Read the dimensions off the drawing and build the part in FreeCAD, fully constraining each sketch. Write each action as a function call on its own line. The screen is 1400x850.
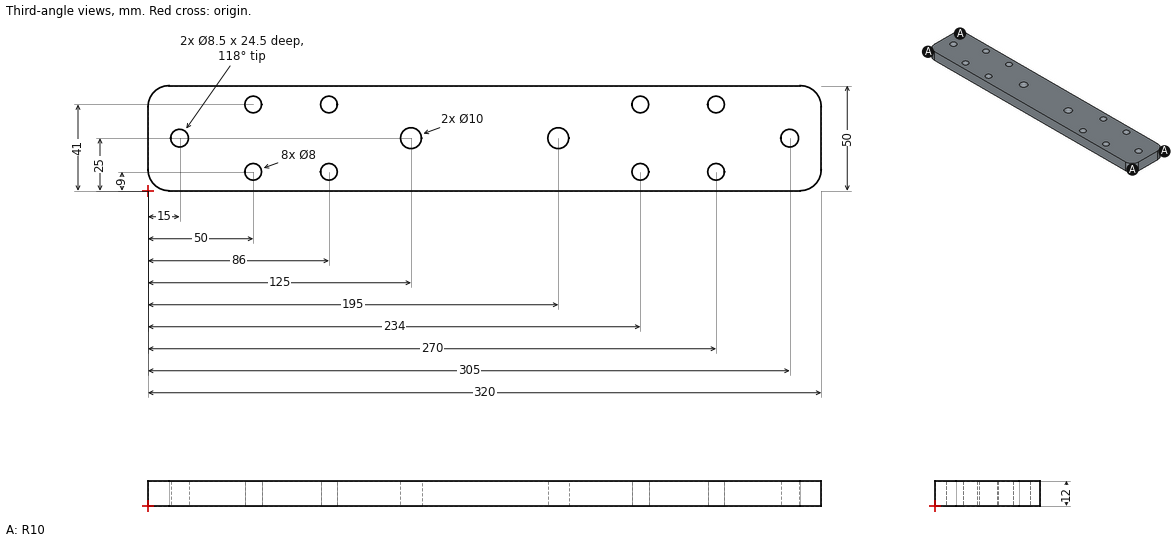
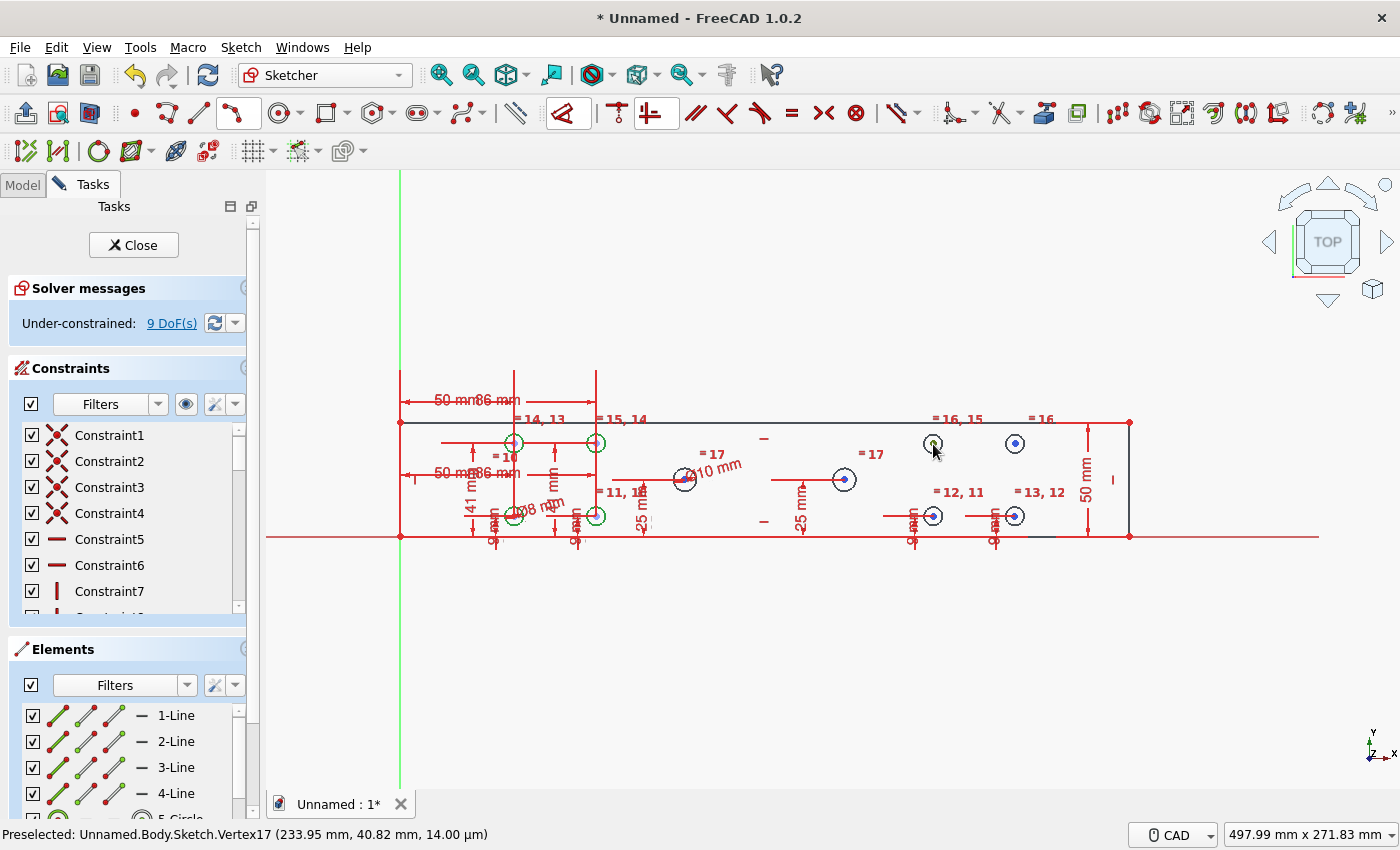
key(i)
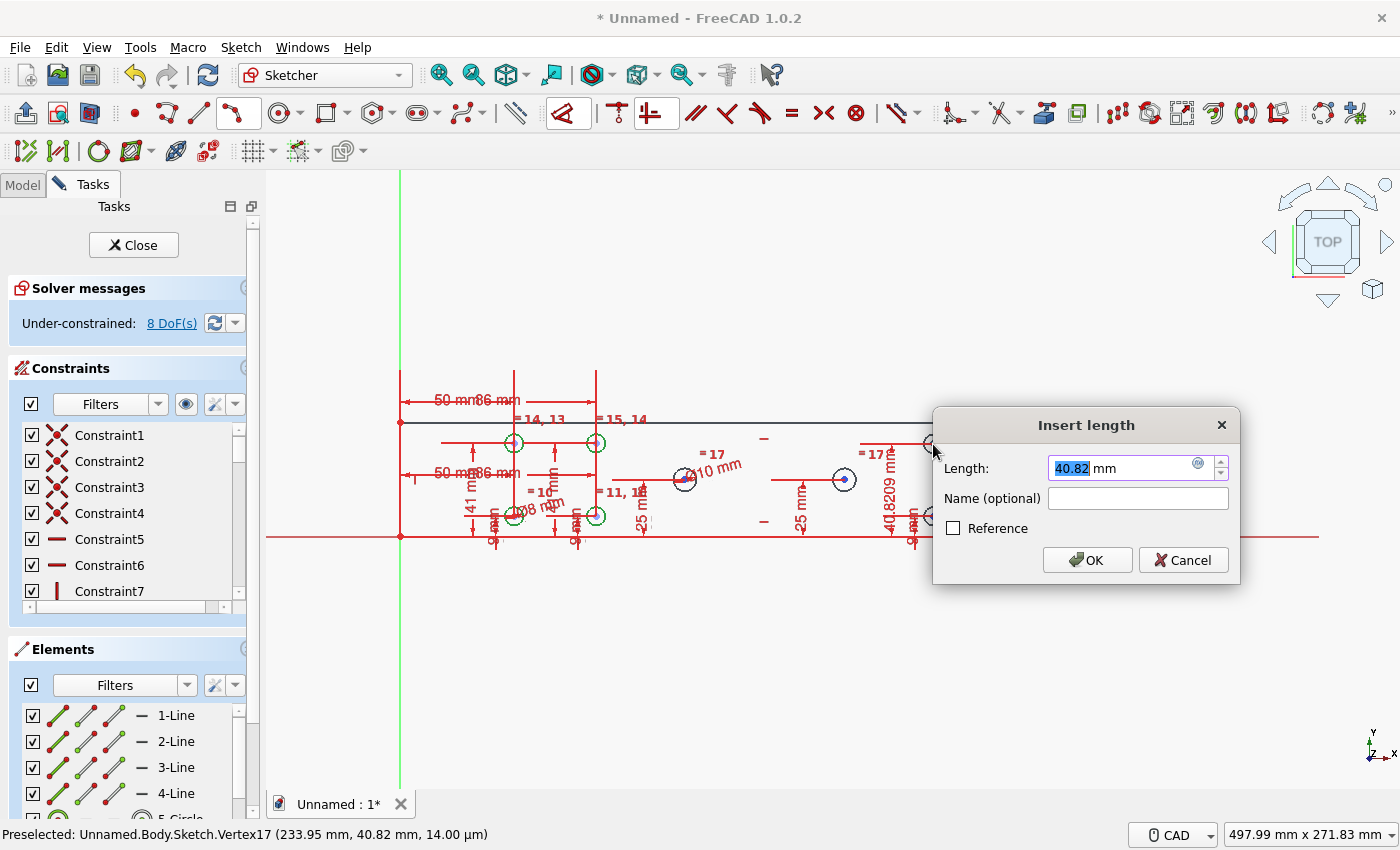
text(41)
key(Return)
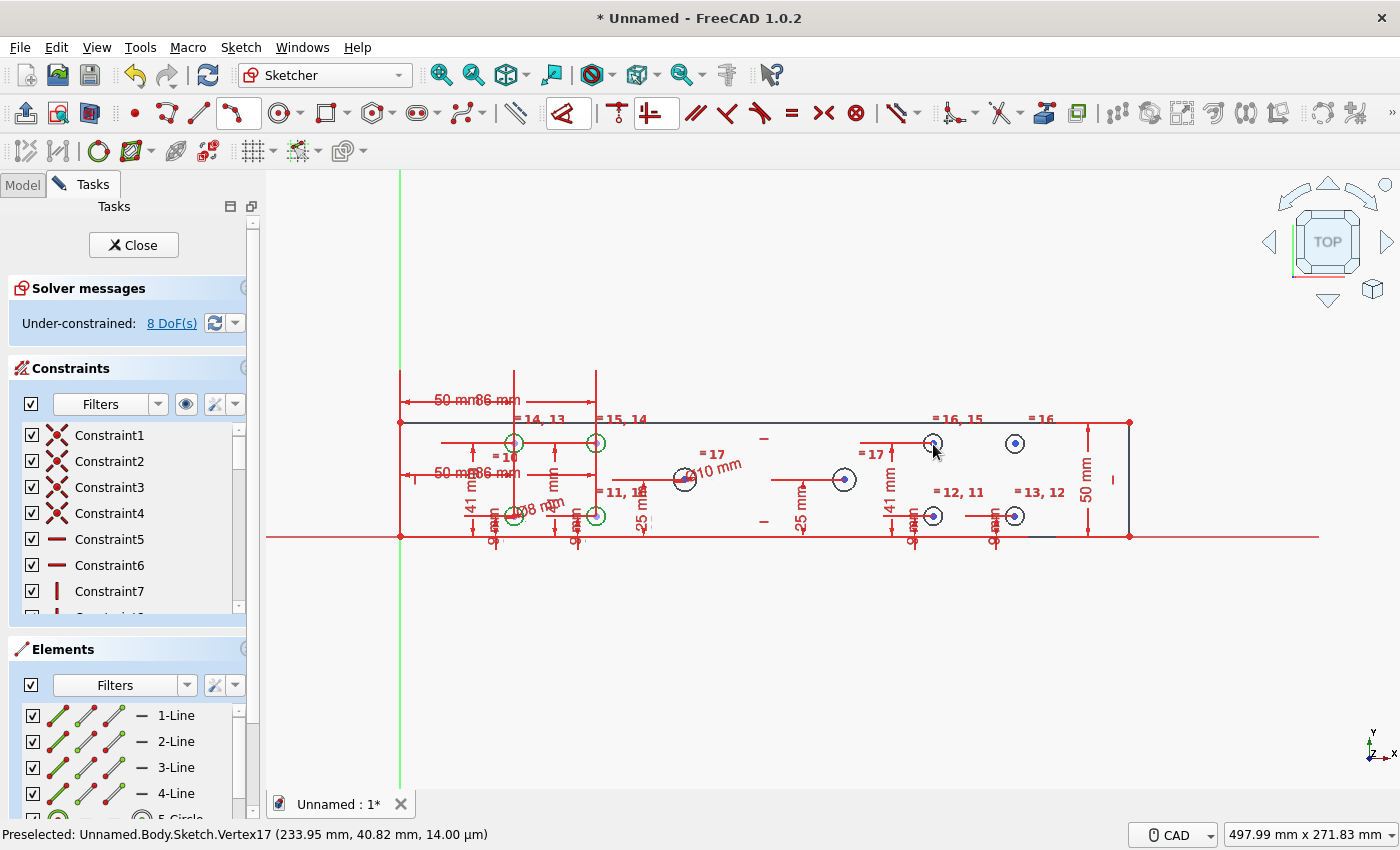
click(1015, 444)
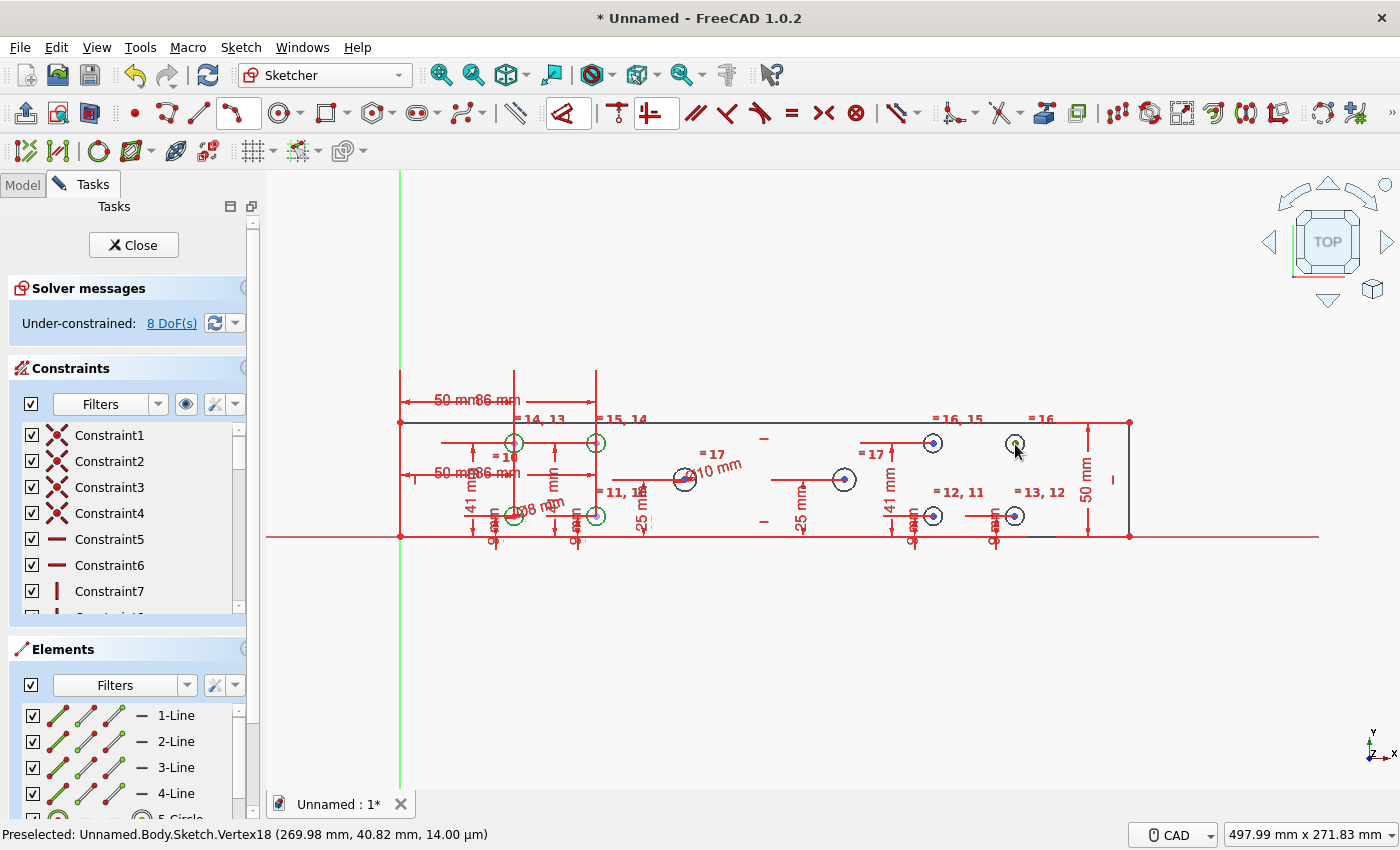
key(i)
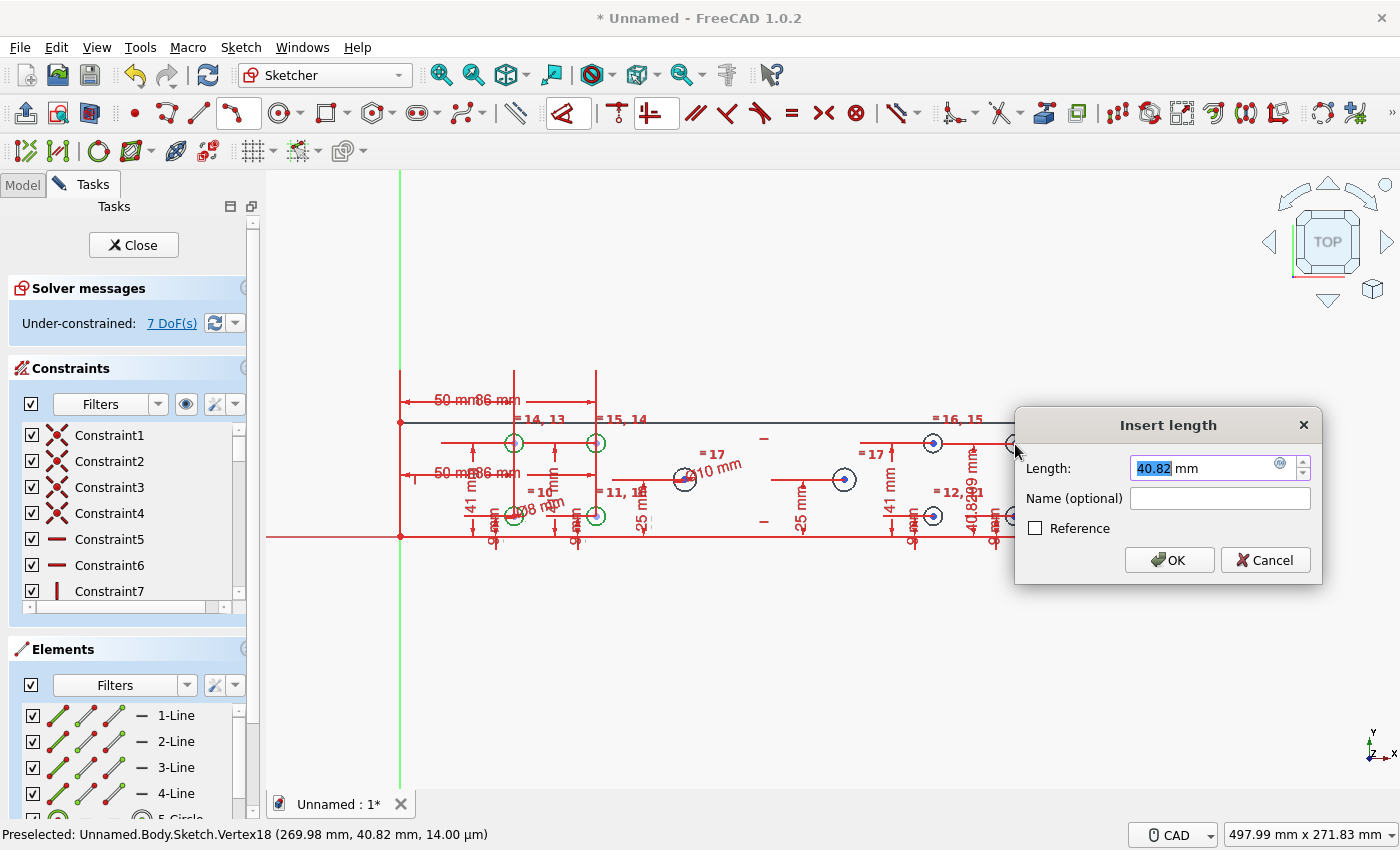
text(41)
key(Return)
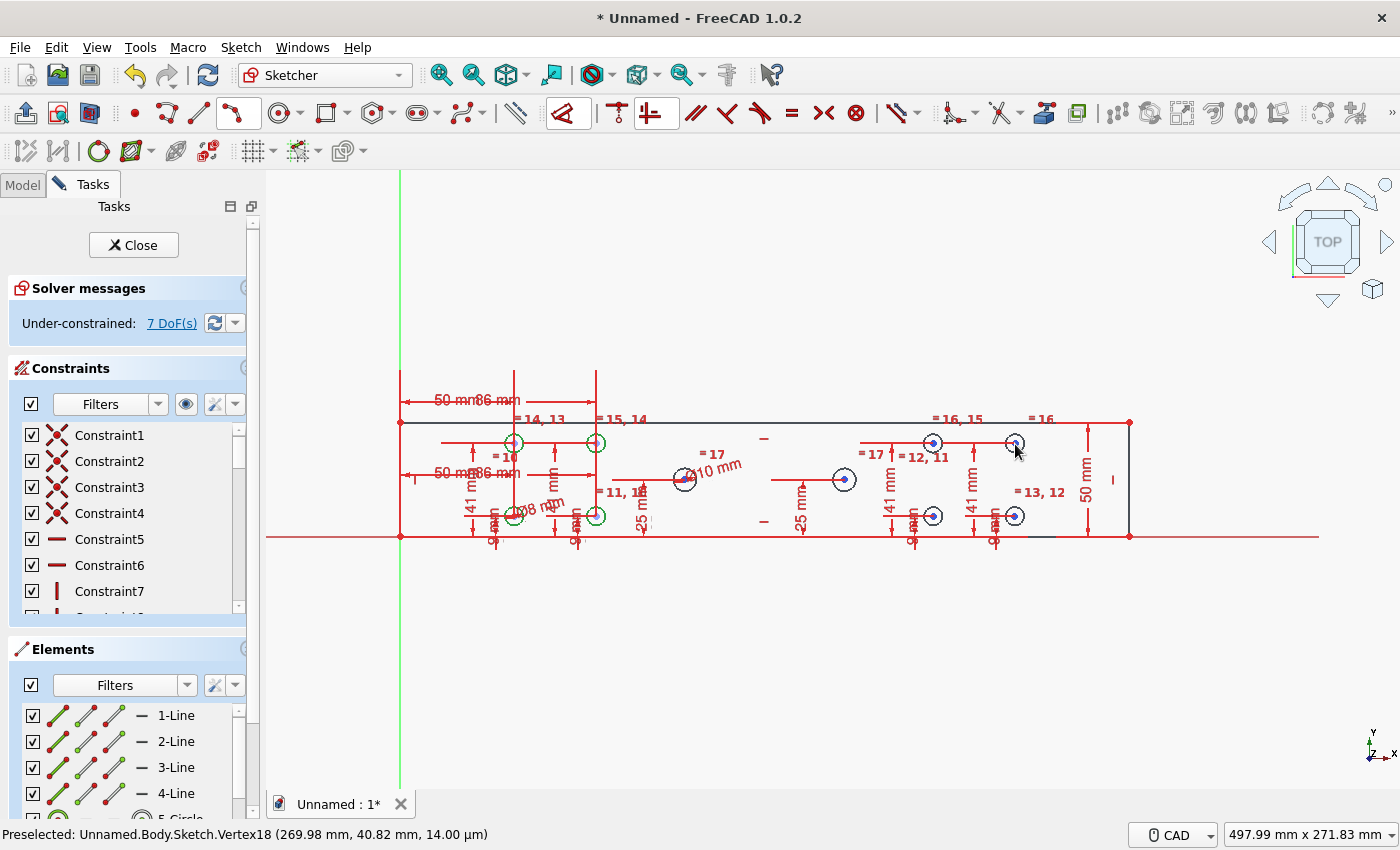
click(619, 537)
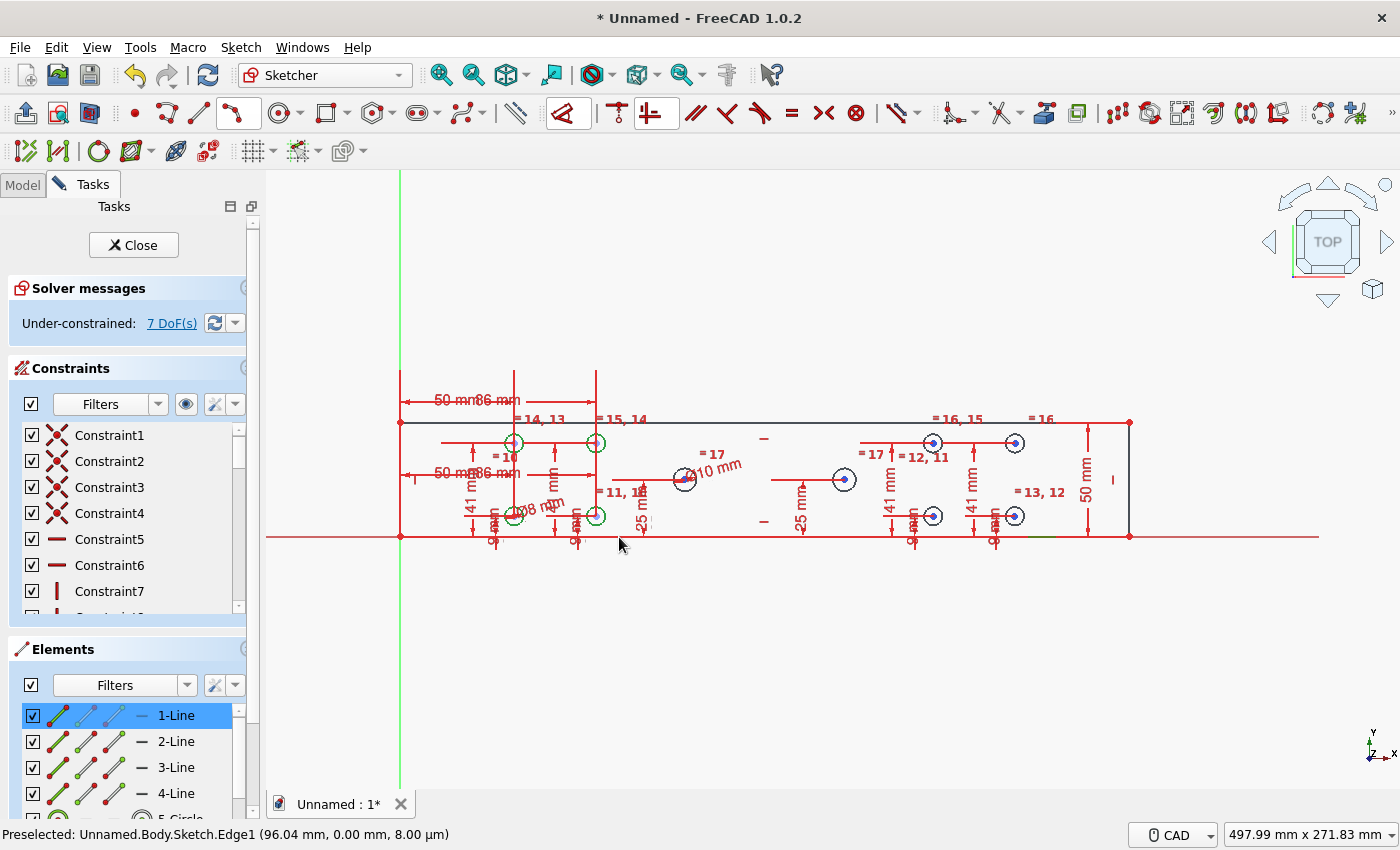
click(586, 114)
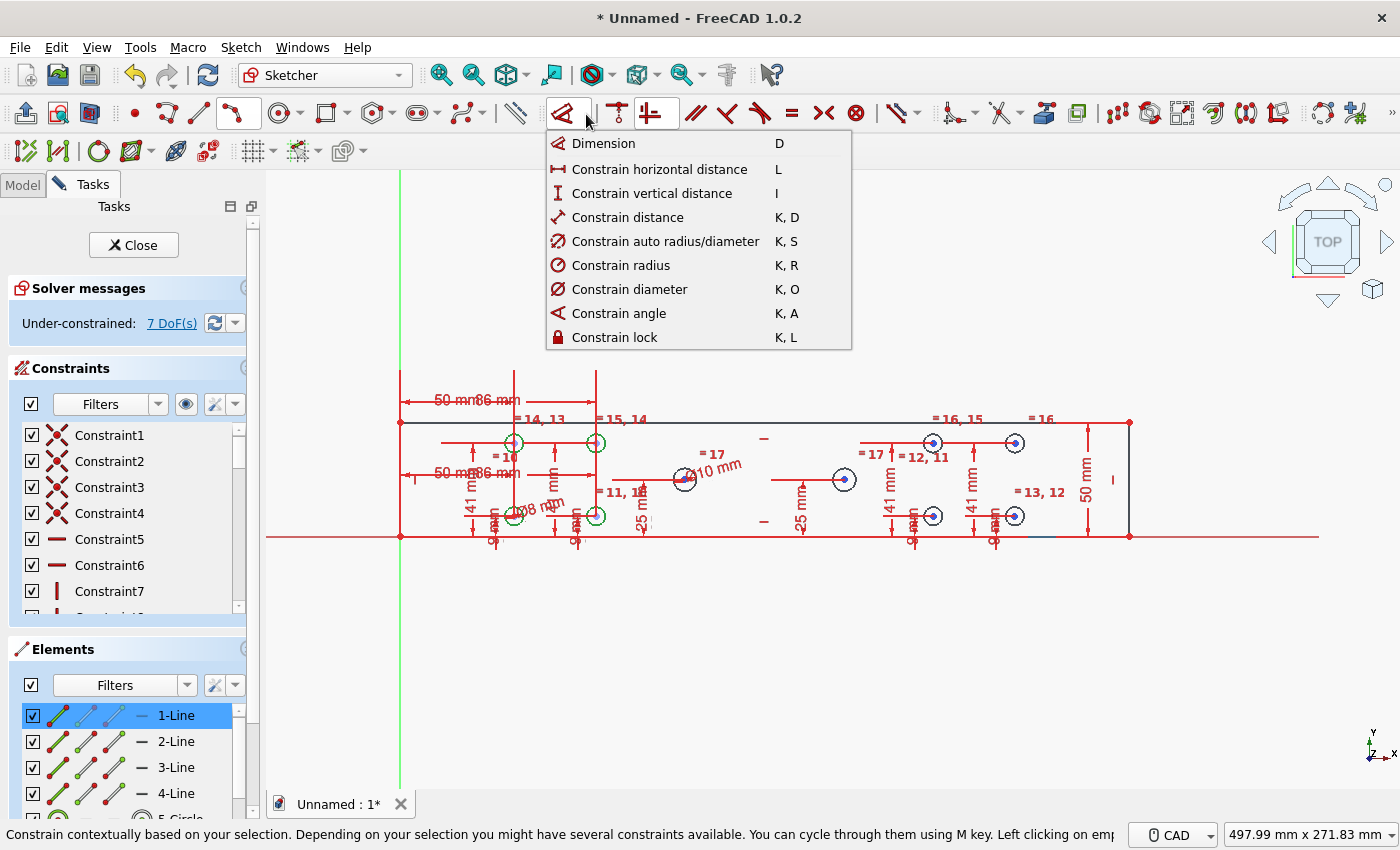
click(699, 169)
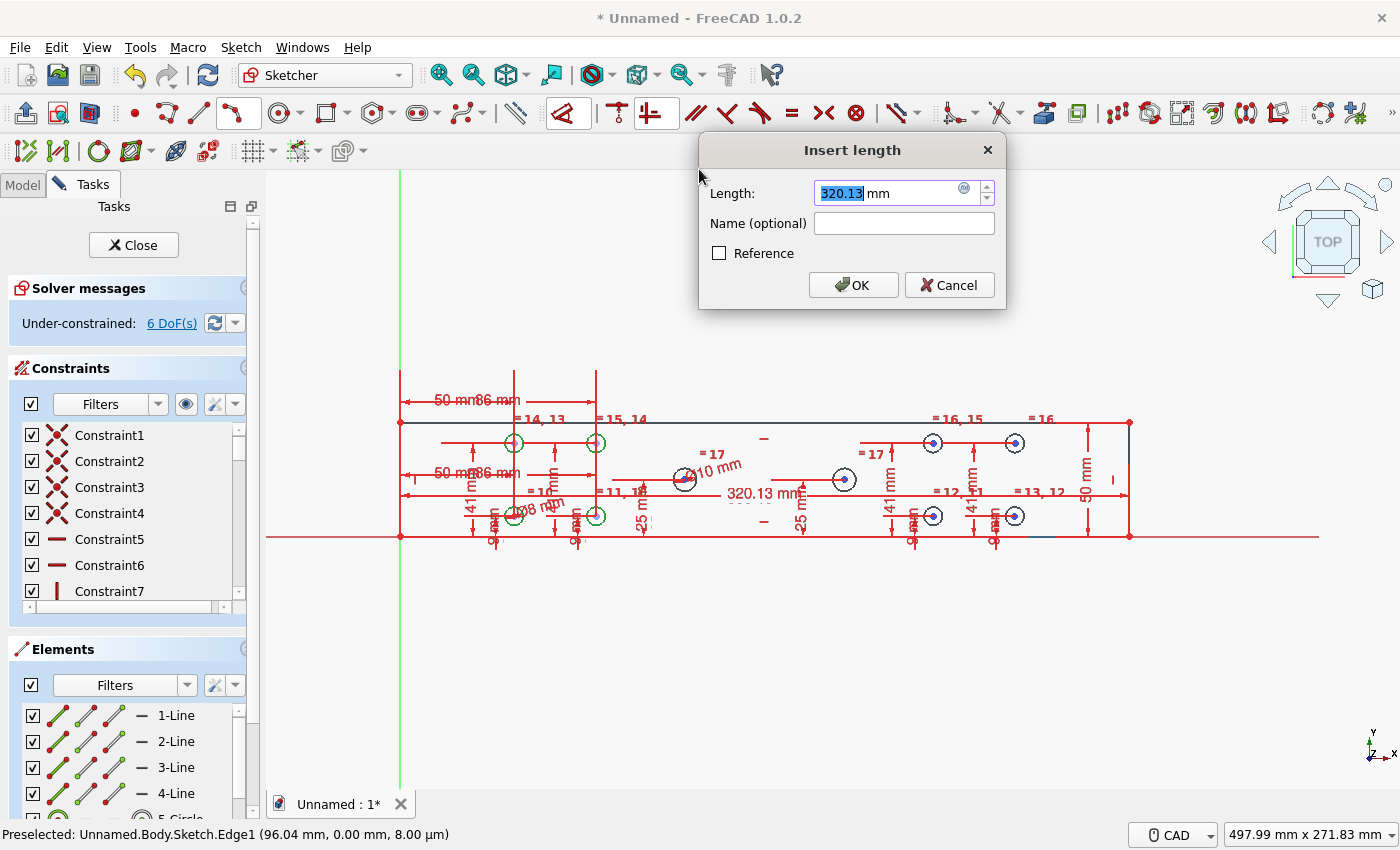
text(320)
key(Return)